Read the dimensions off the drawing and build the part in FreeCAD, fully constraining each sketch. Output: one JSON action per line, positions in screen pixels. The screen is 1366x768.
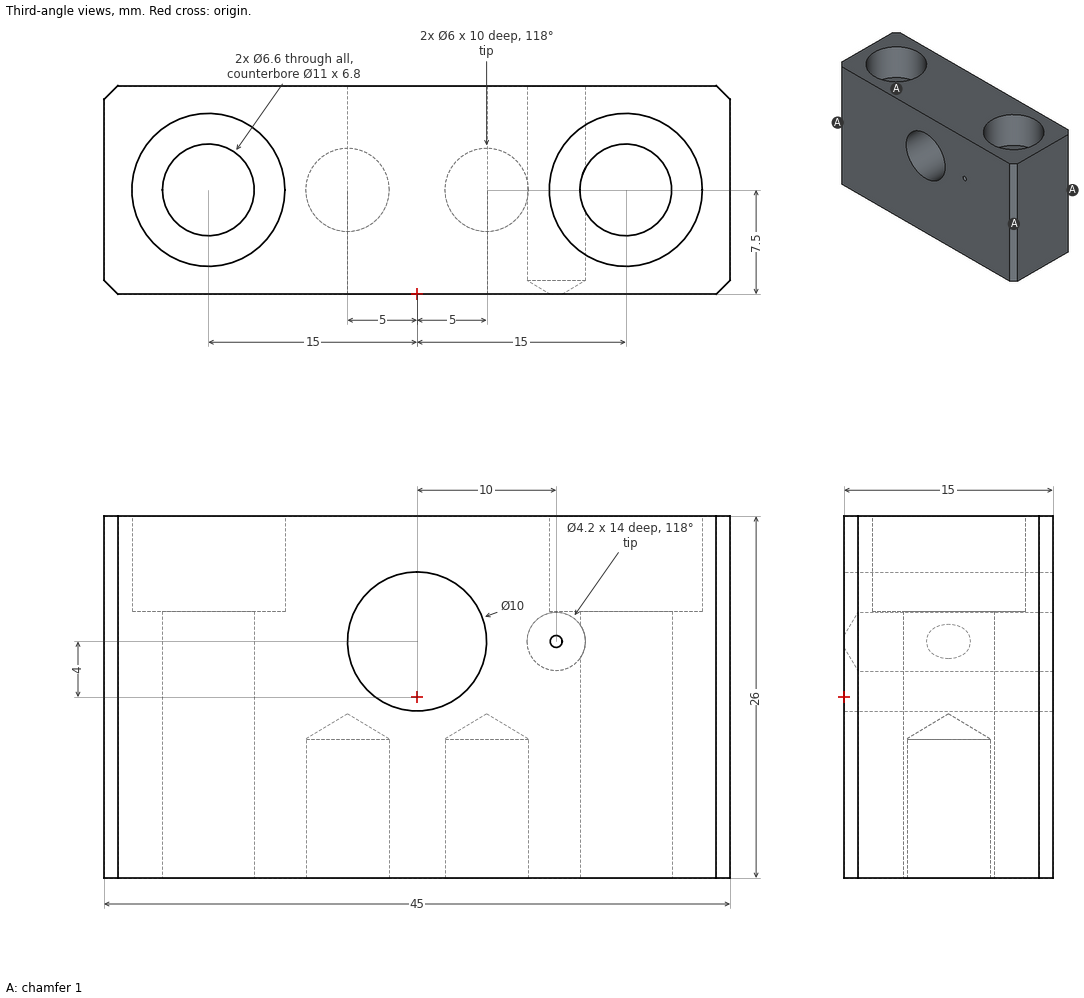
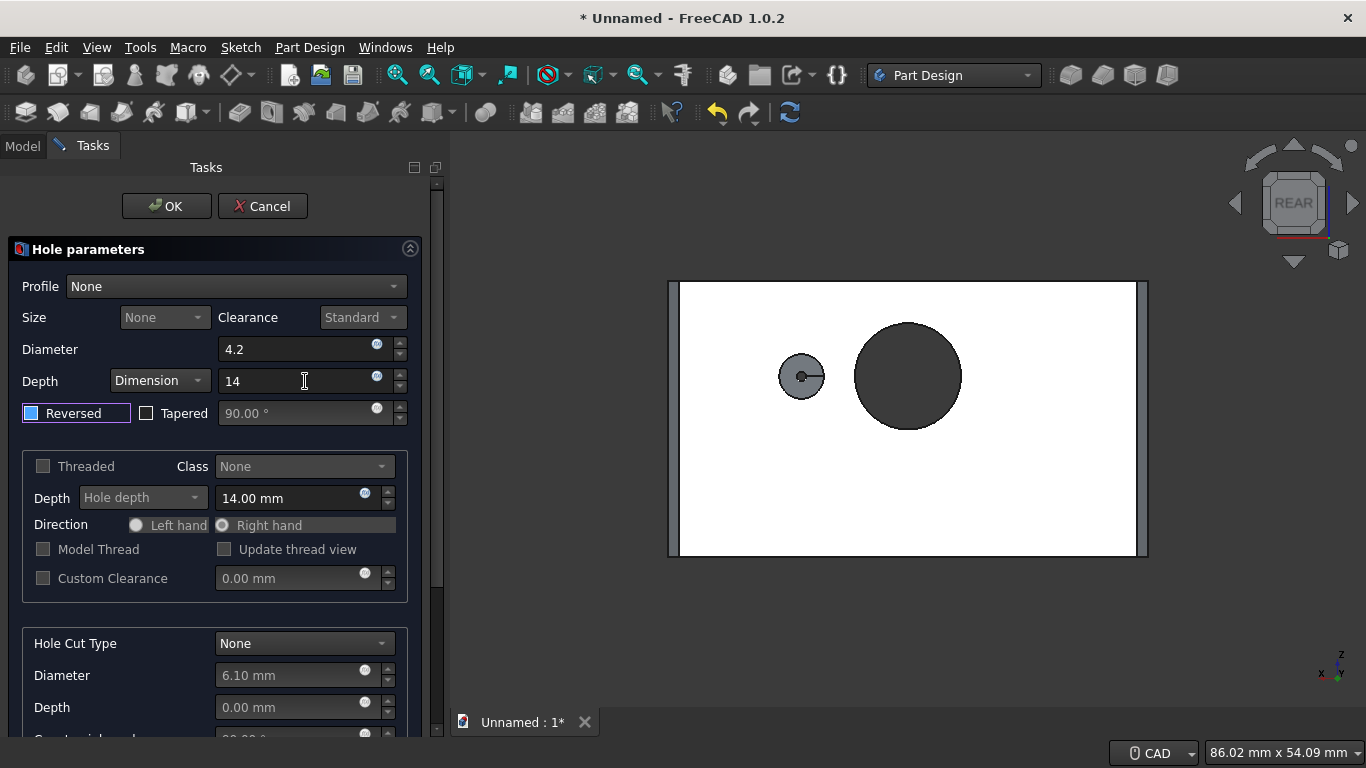
{"action": "left_click", "coordinate": [167, 206]}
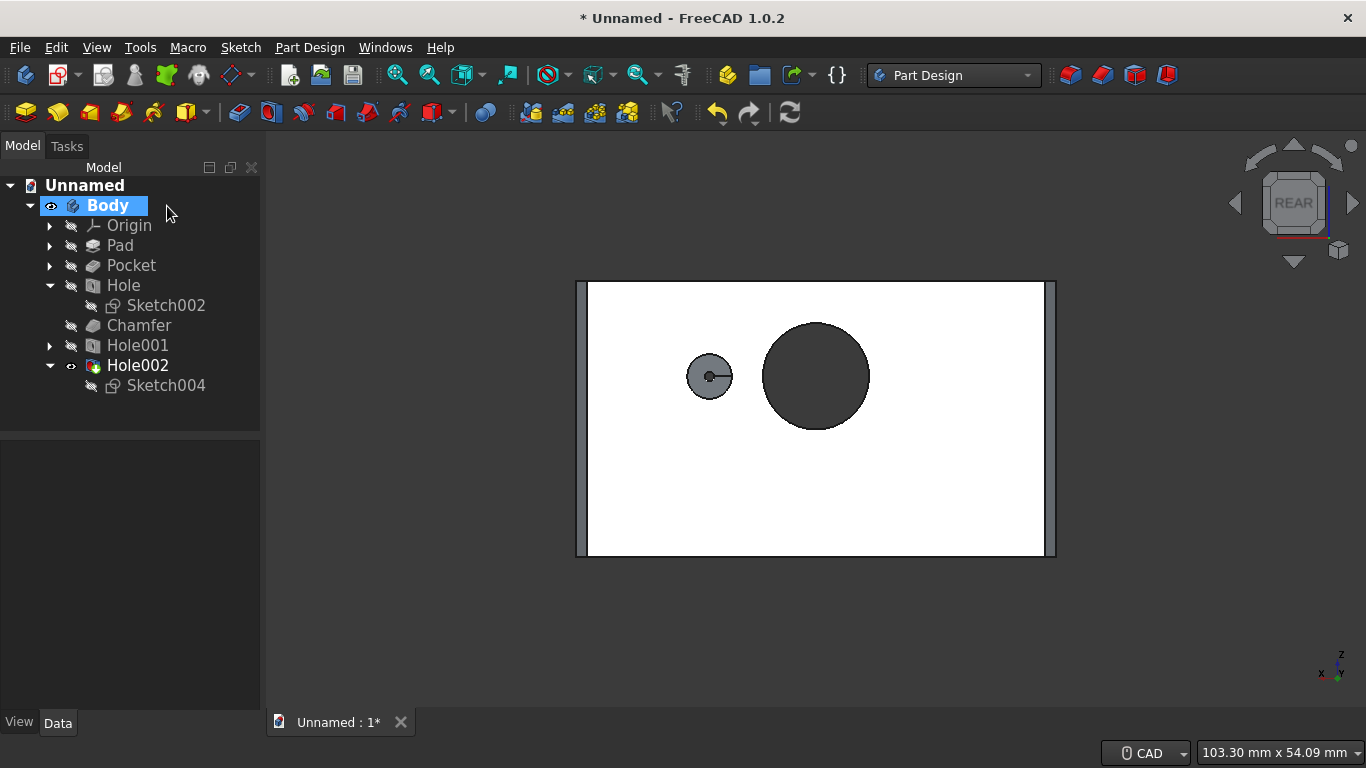
{"action": "key", "text": "0"}